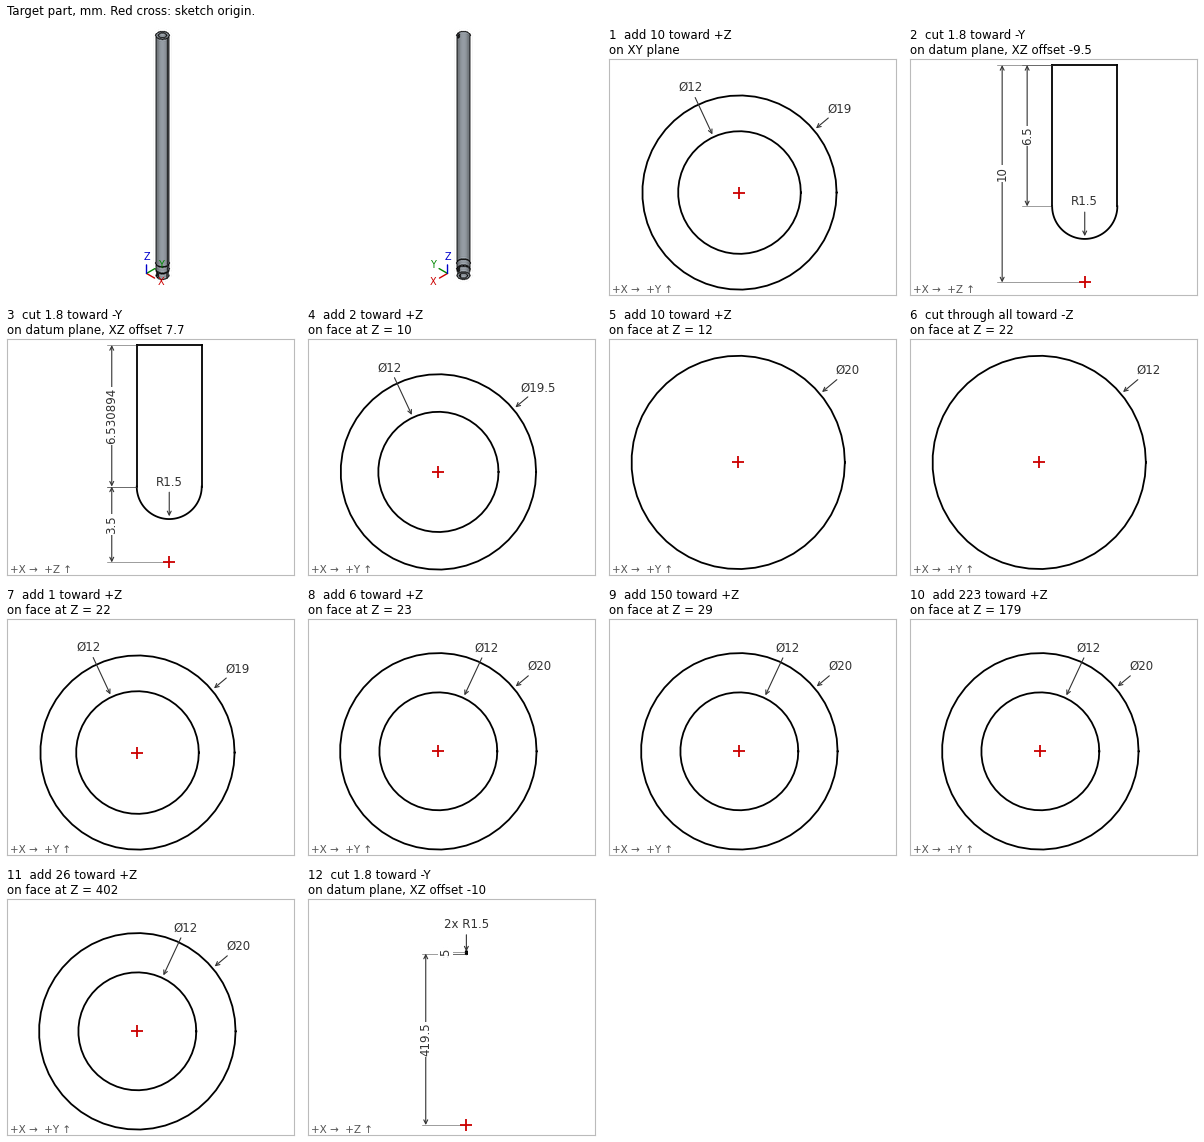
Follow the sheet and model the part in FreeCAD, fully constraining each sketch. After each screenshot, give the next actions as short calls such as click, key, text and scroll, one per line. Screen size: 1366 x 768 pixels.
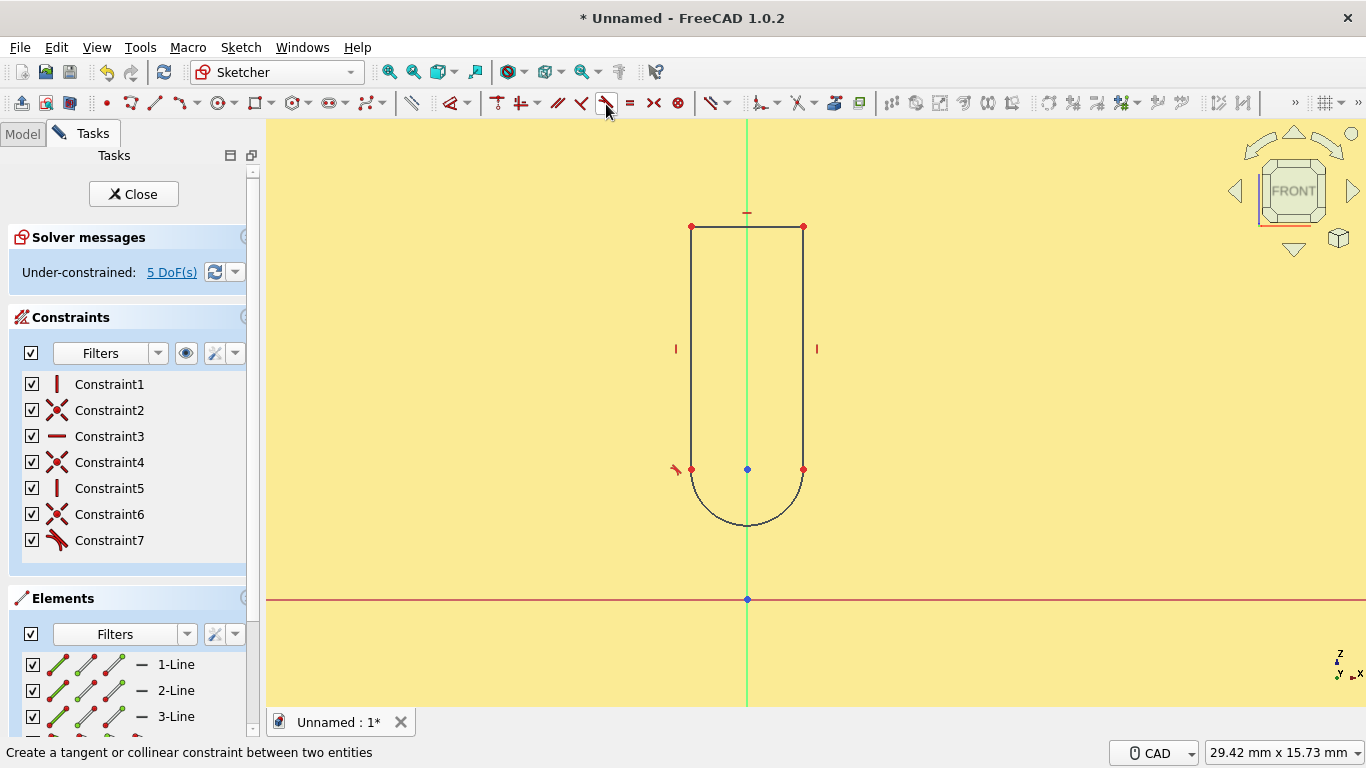
click(803, 300)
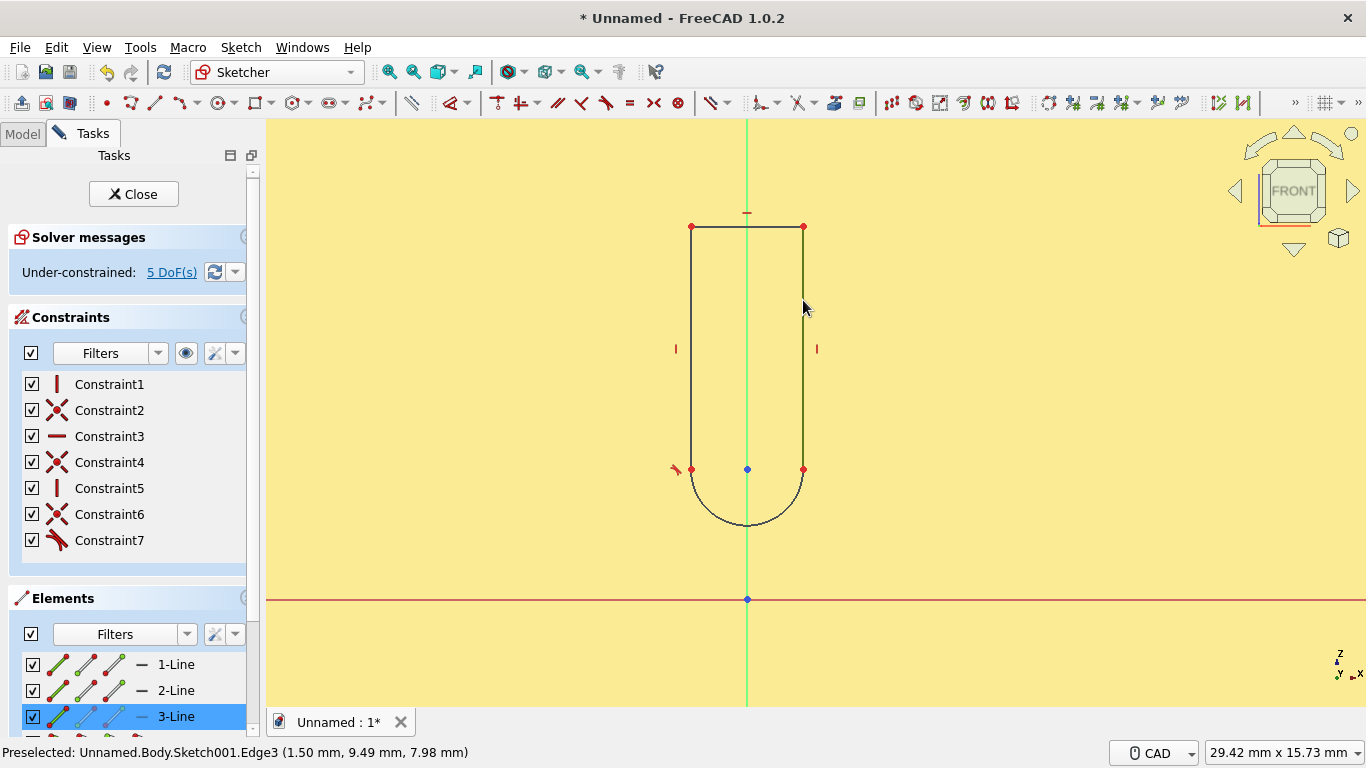
click(714, 515)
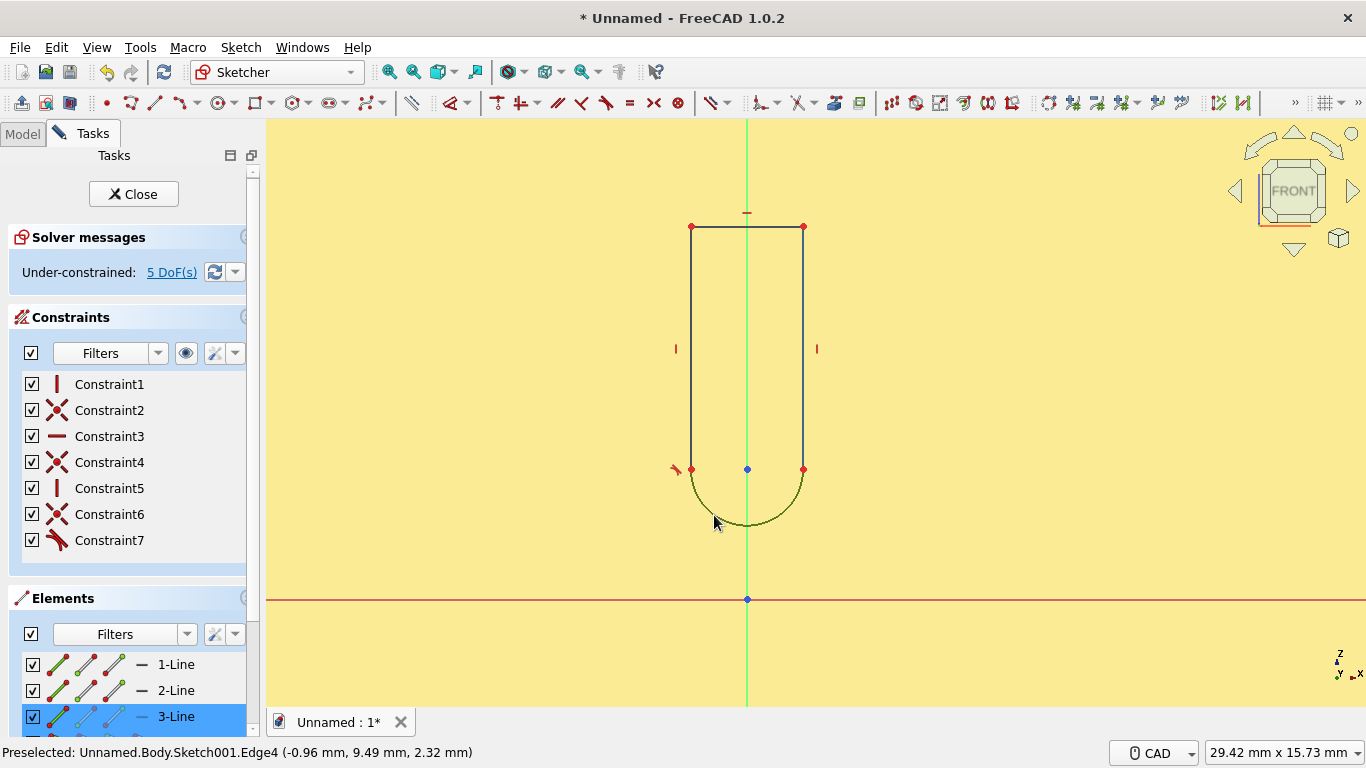
click(606, 104)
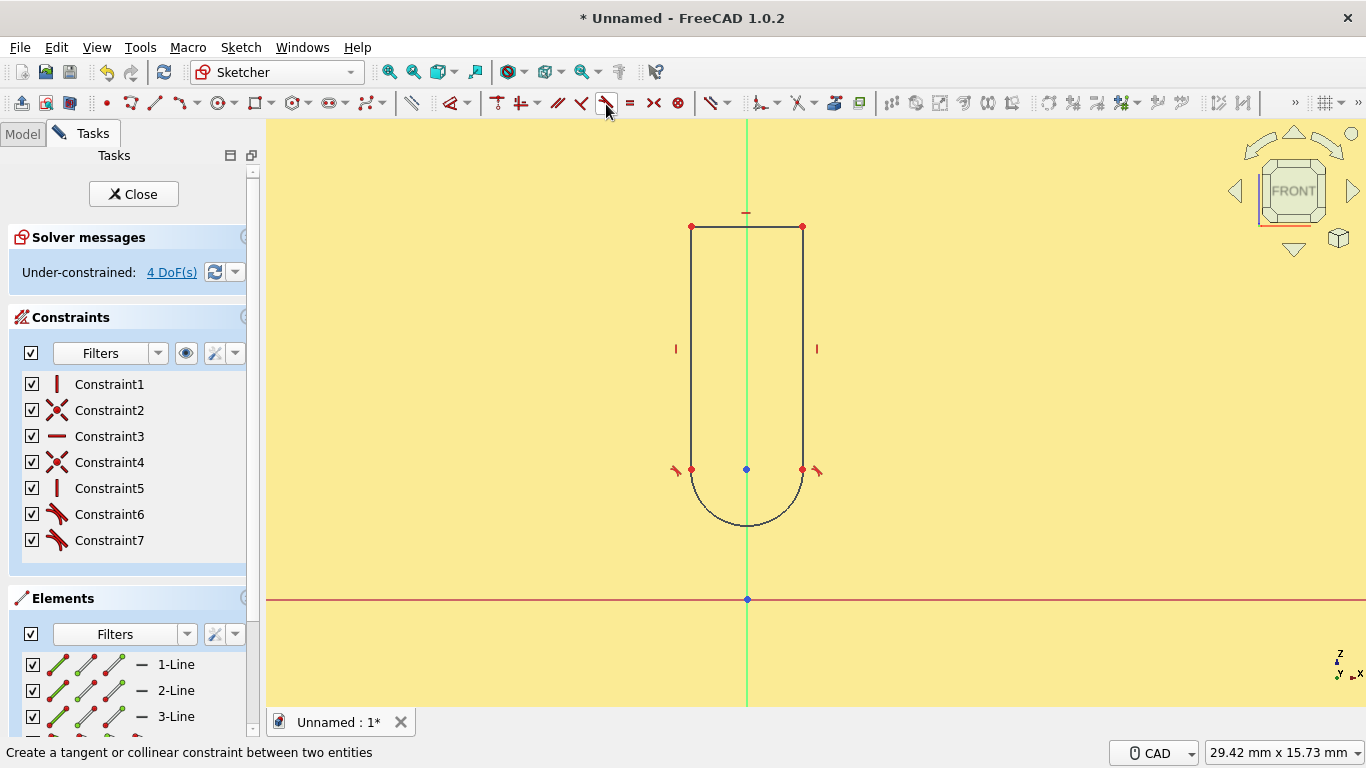
click(747, 470)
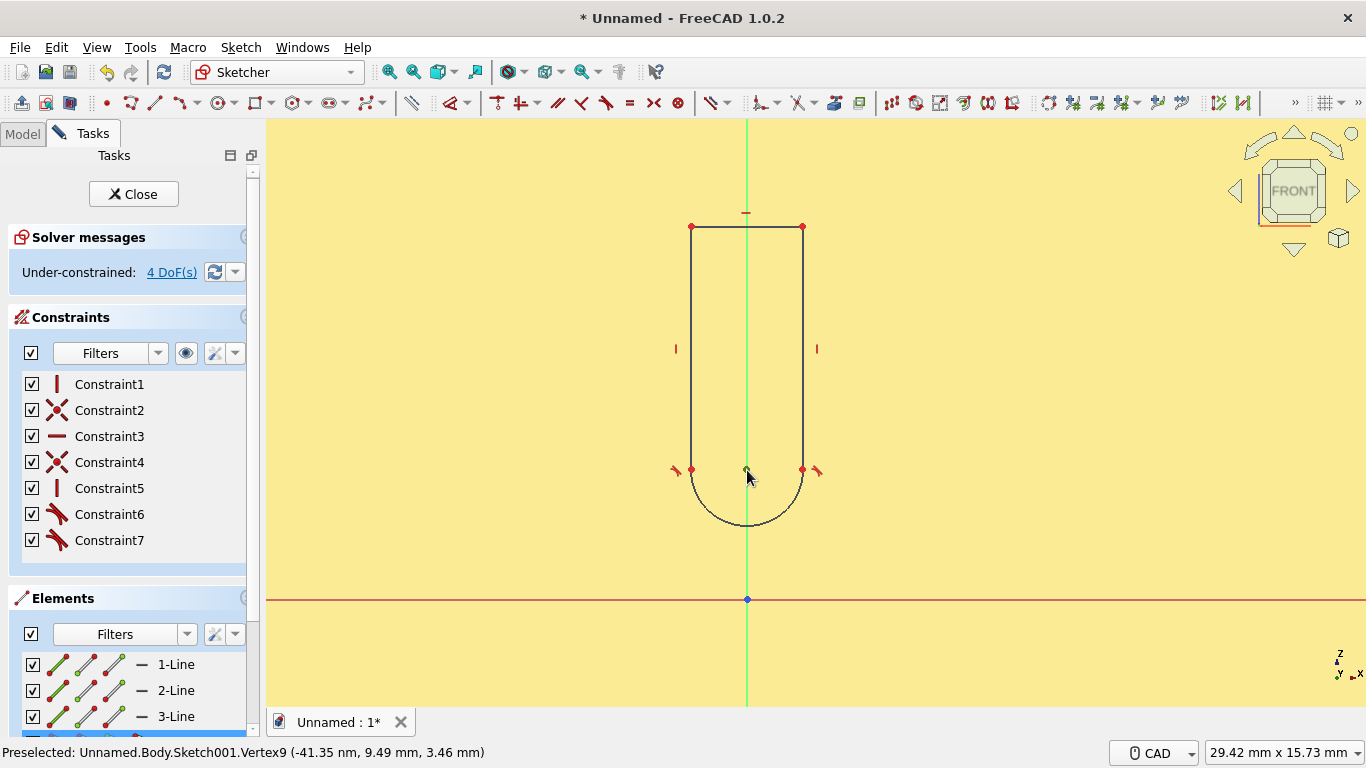
click(747, 641)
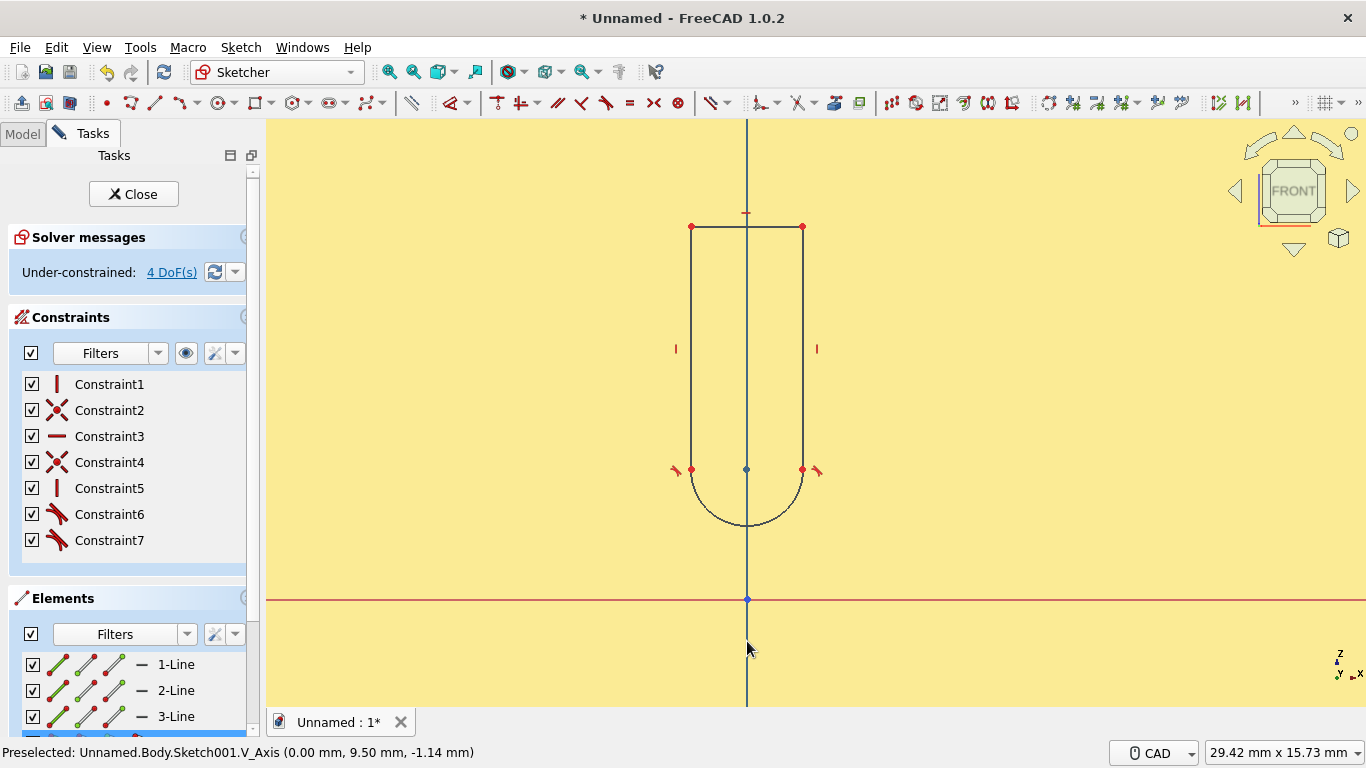
click(498, 104)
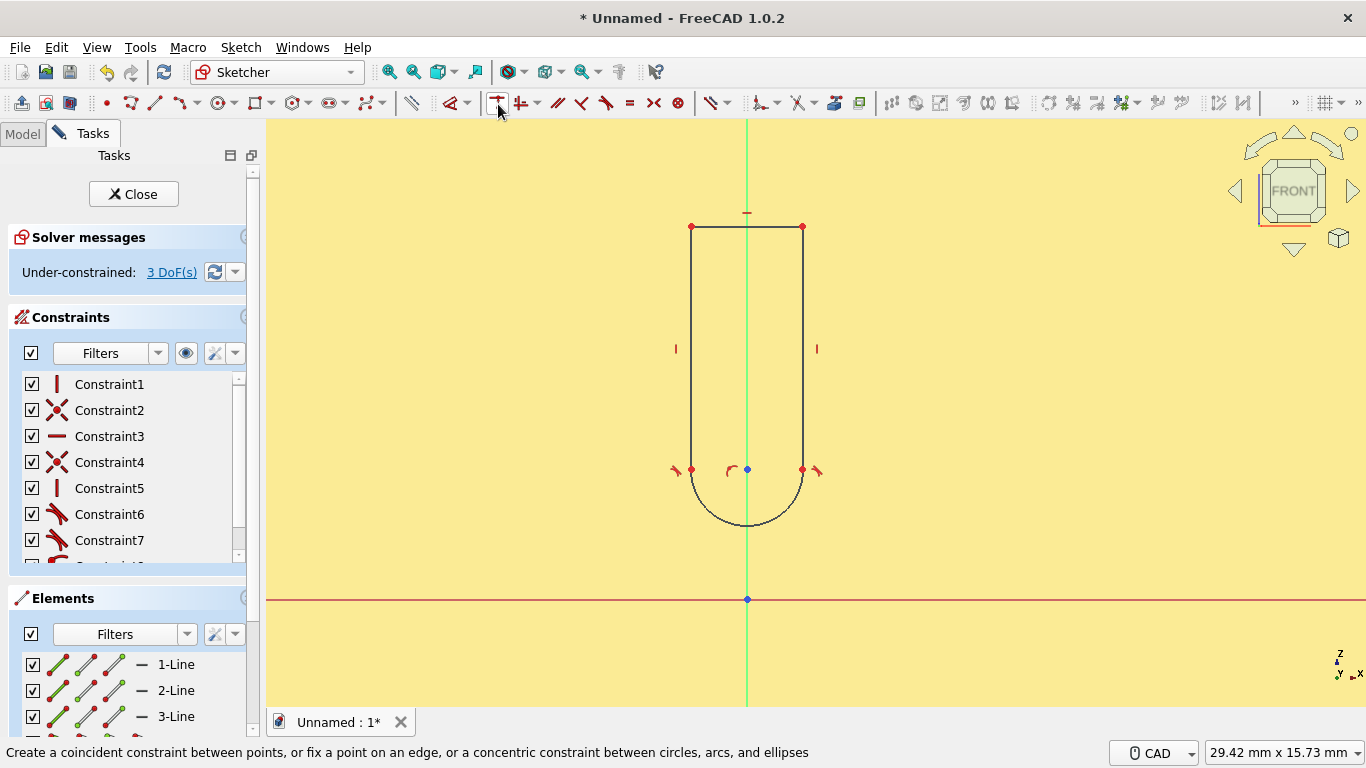
click(450, 104)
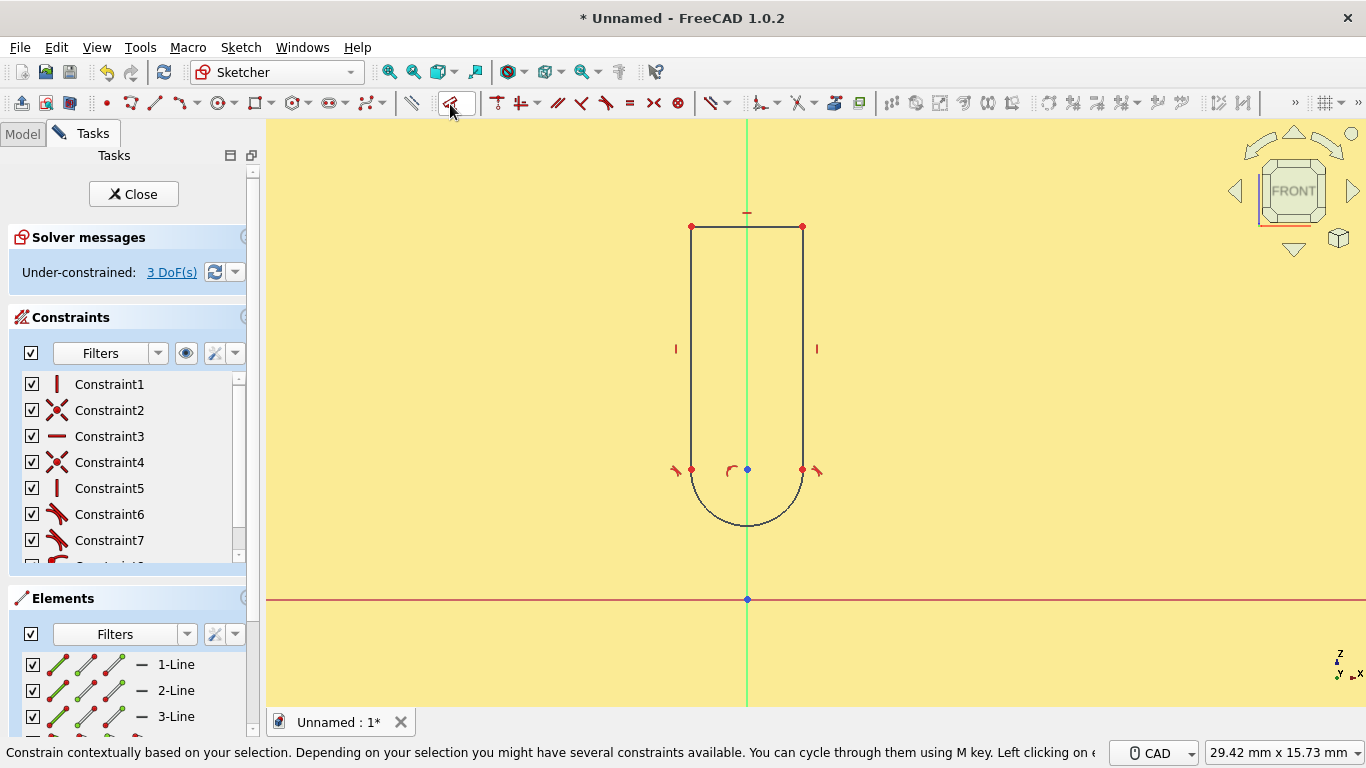
click(714, 515)
click(695, 541)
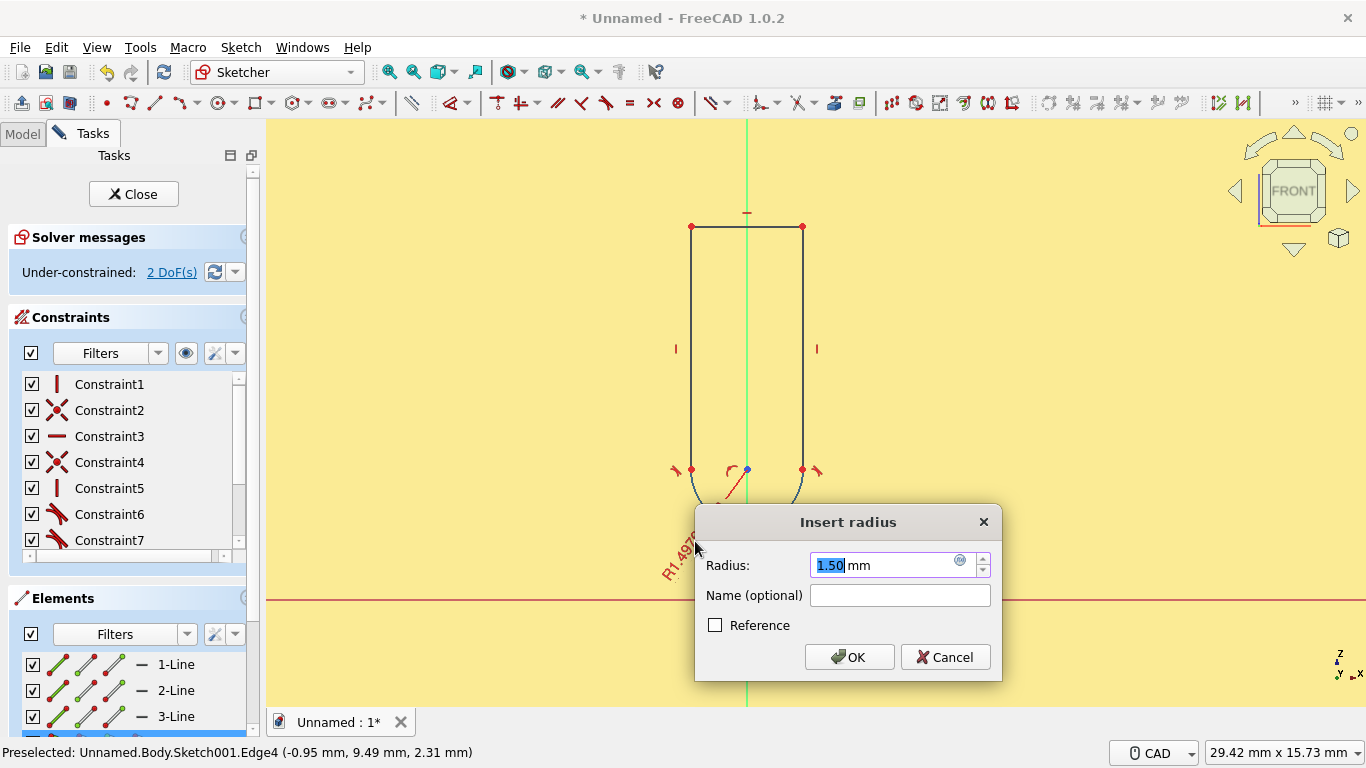
text(1.5)
key(Return)